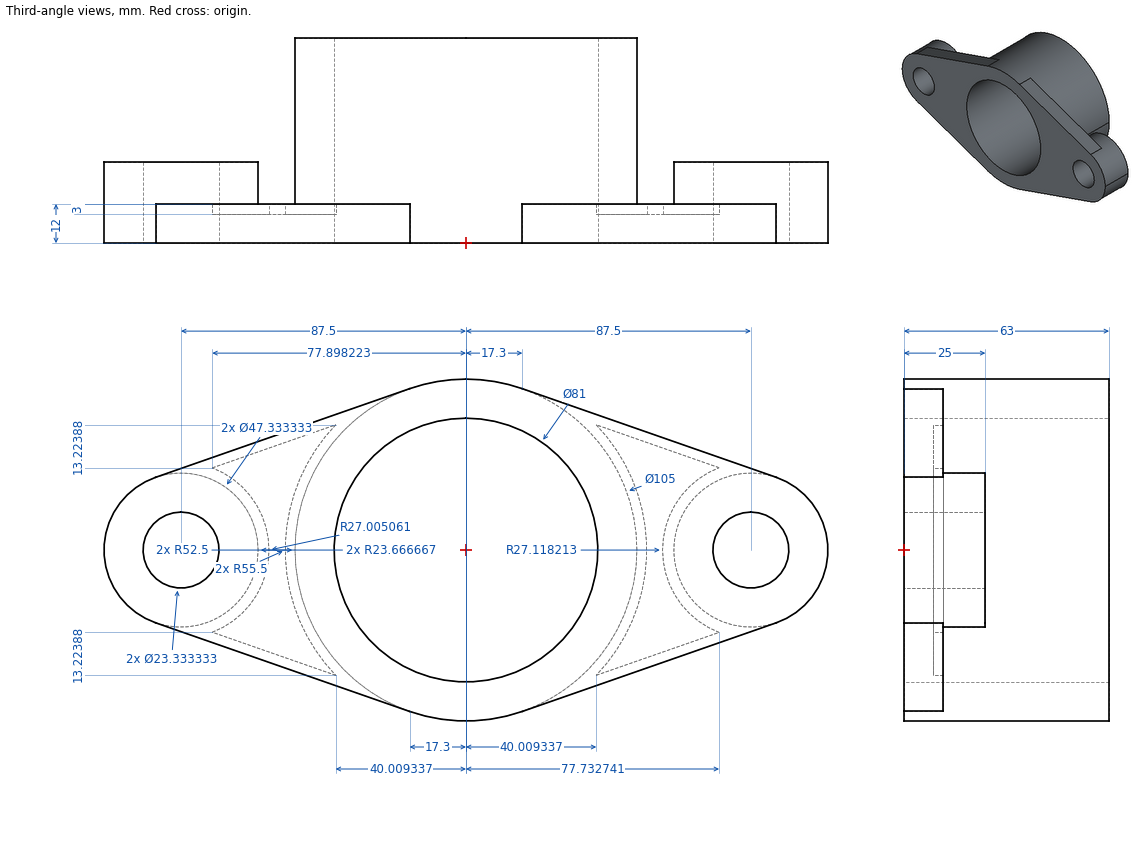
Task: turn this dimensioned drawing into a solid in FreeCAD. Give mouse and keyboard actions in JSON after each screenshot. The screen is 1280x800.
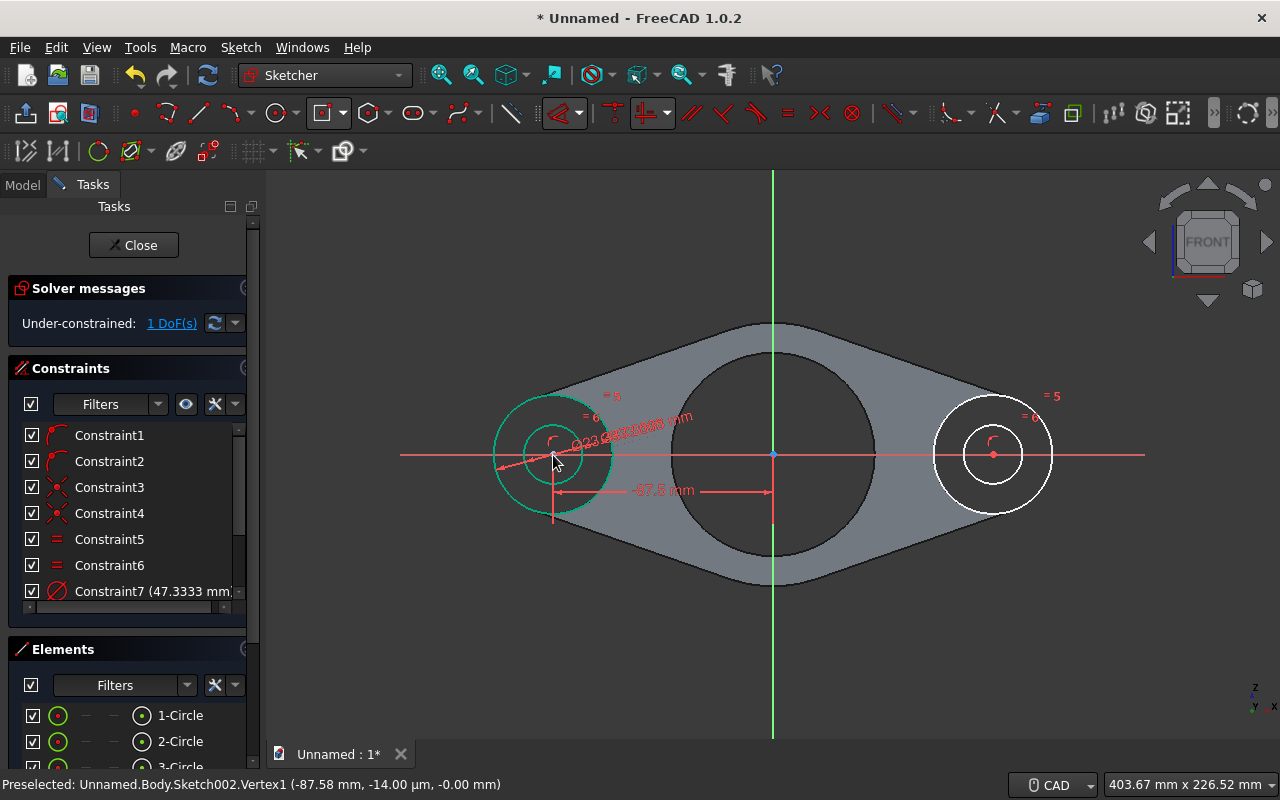
{"action": "left_click", "coordinate": [993, 455]}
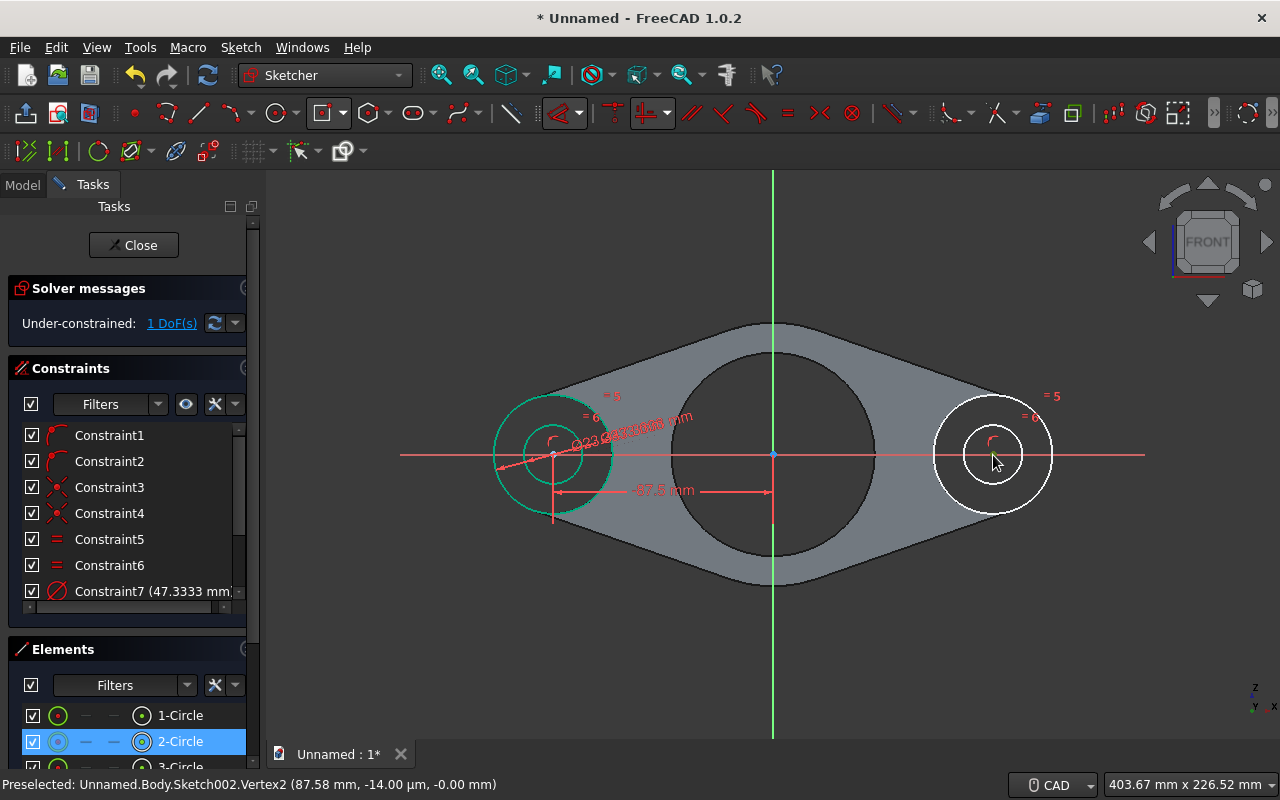
{"action": "key", "text": "l"}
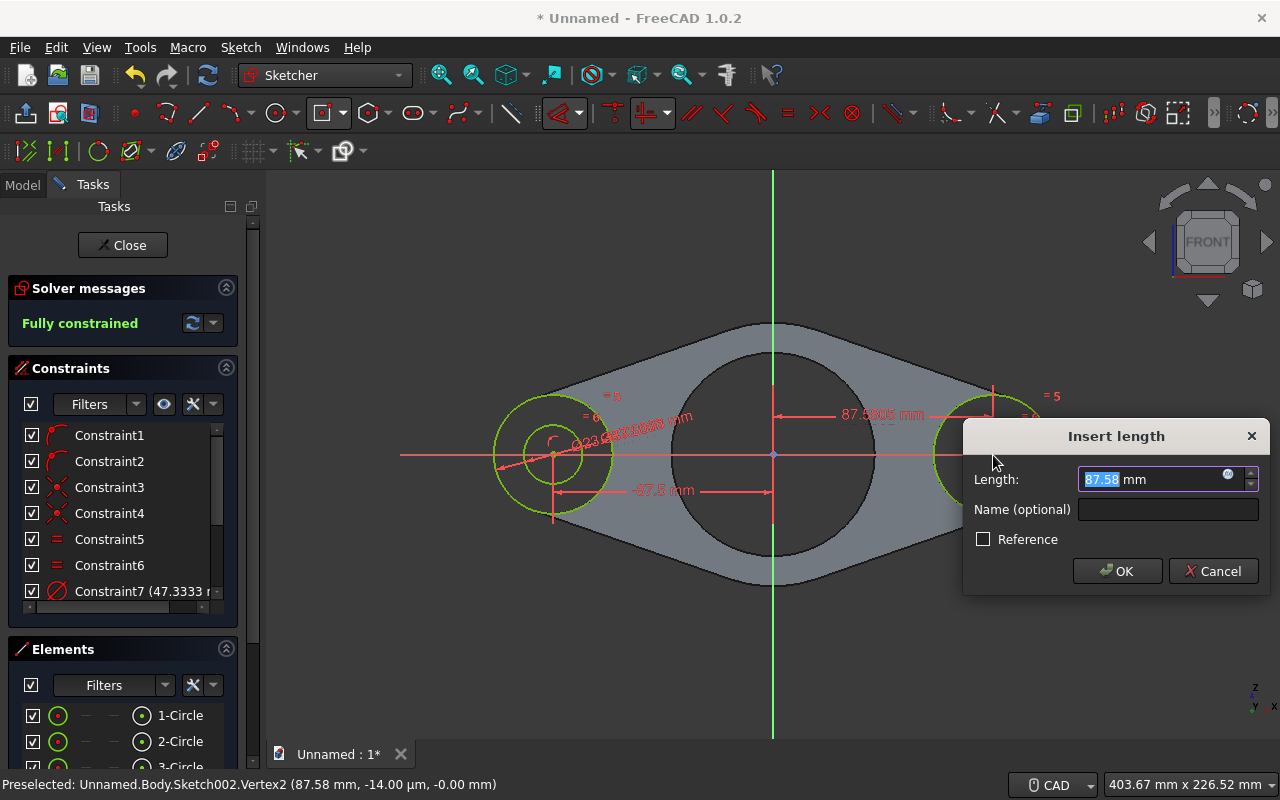
{"action": "type", "text": "87.5"}
{"action": "key", "text": "Return"}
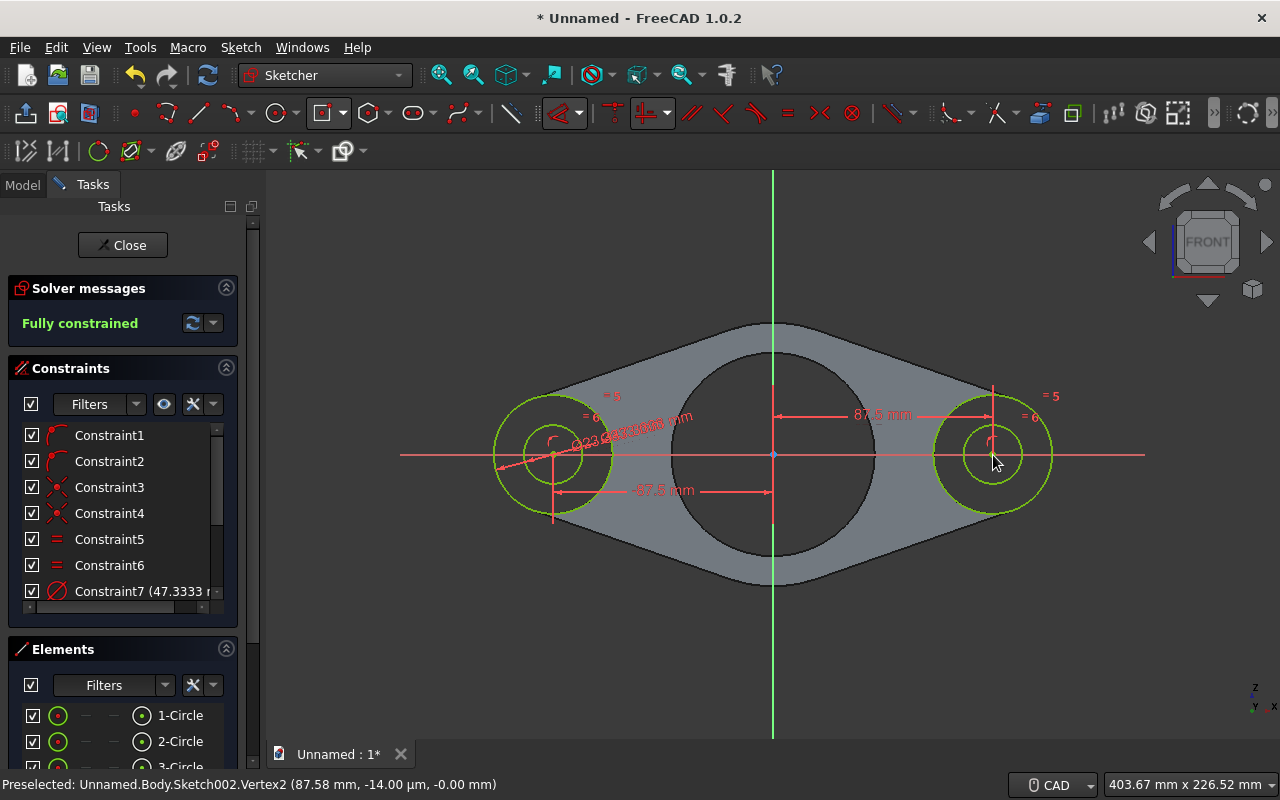
{"action": "left_click", "coordinate": [123, 245]}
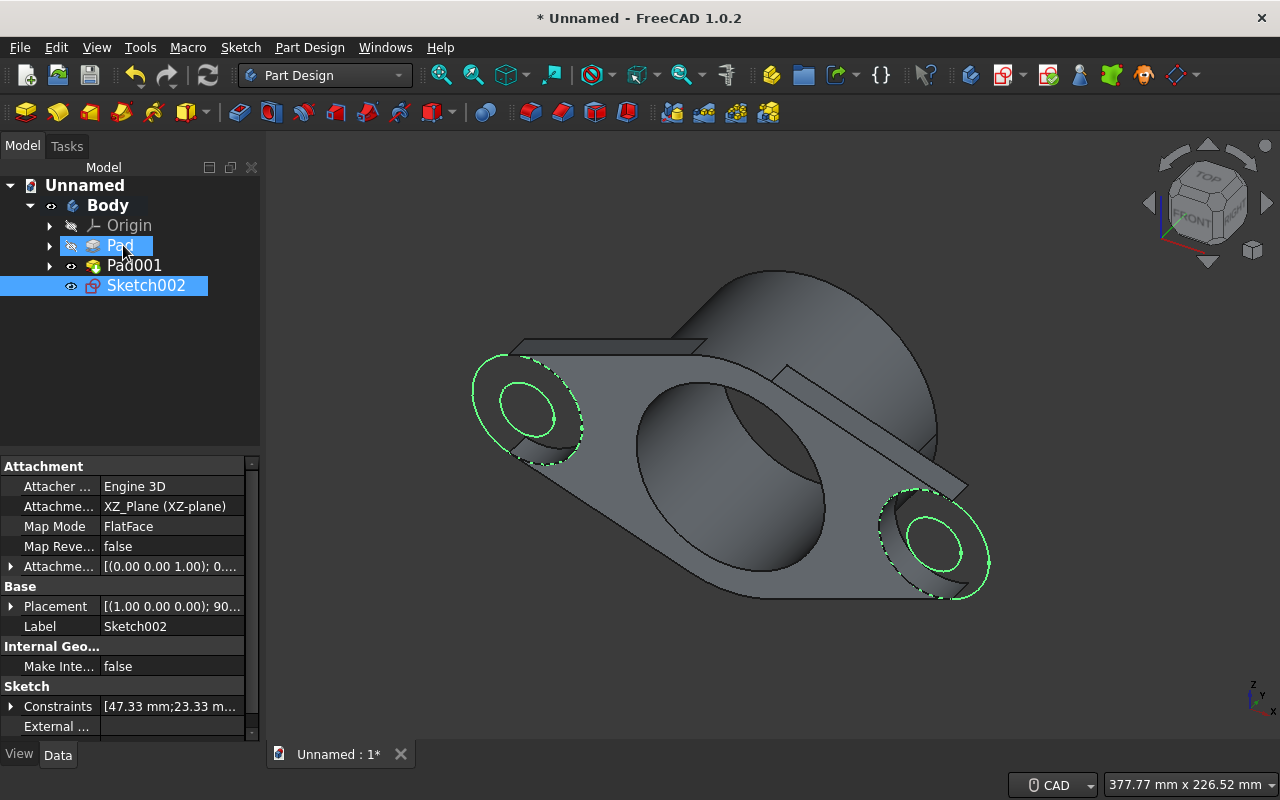
{"action": "left_click", "coordinate": [26, 112]}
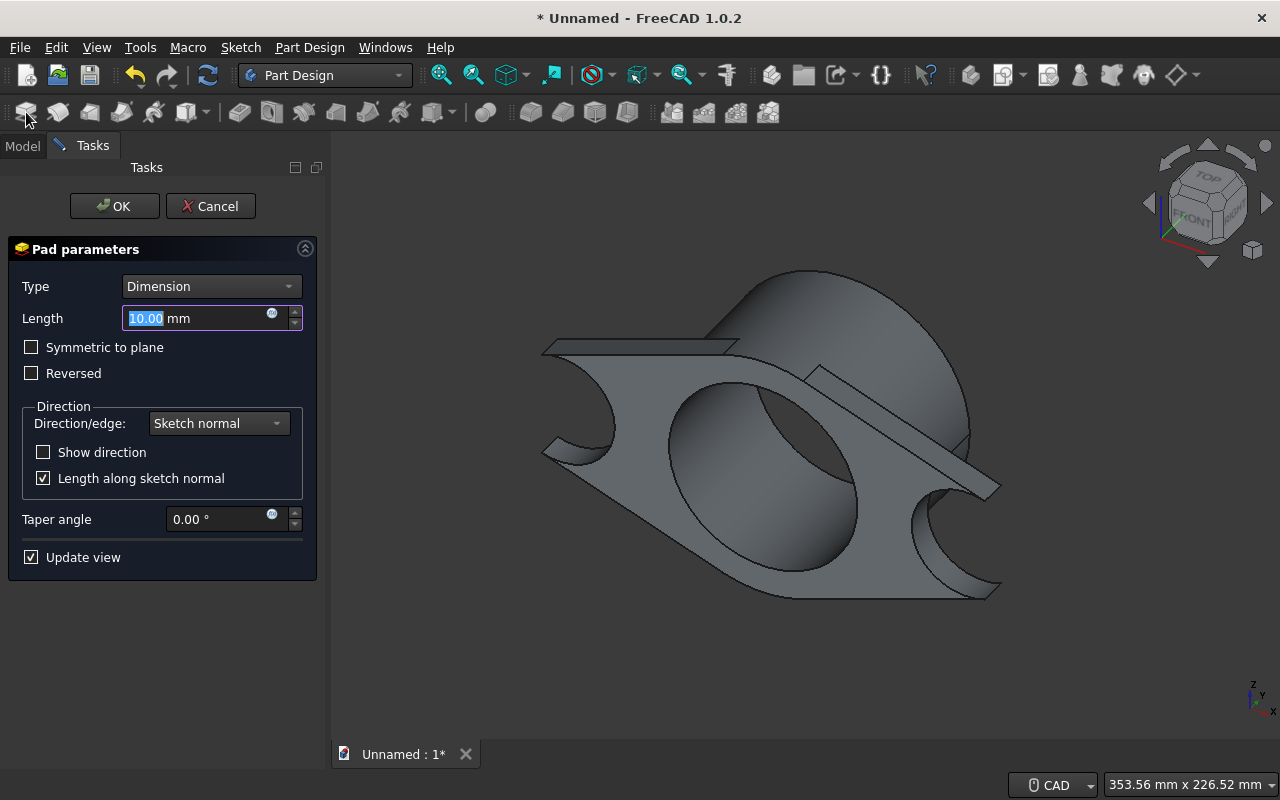
{"action": "type", "text": "25"}
{"action": "key", "text": "Tab"}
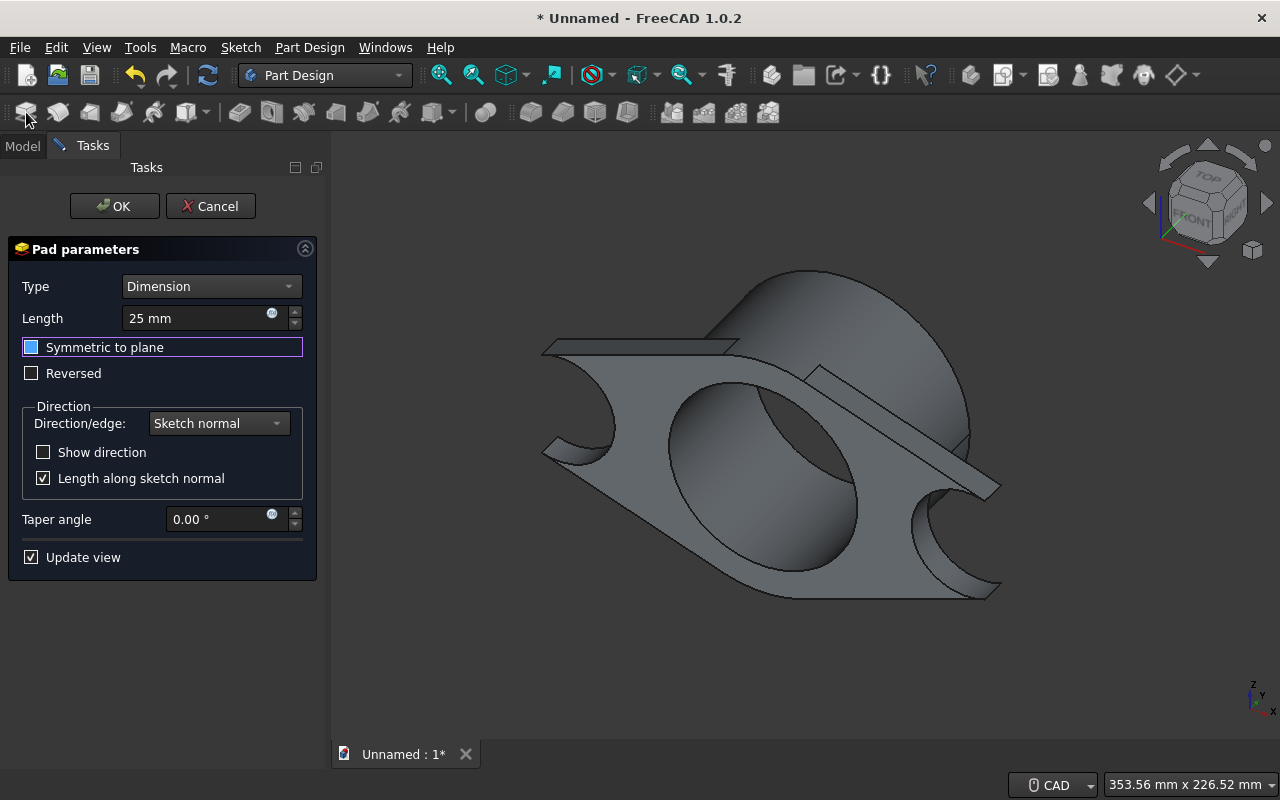
{"action": "left_click", "coordinate": [30, 373]}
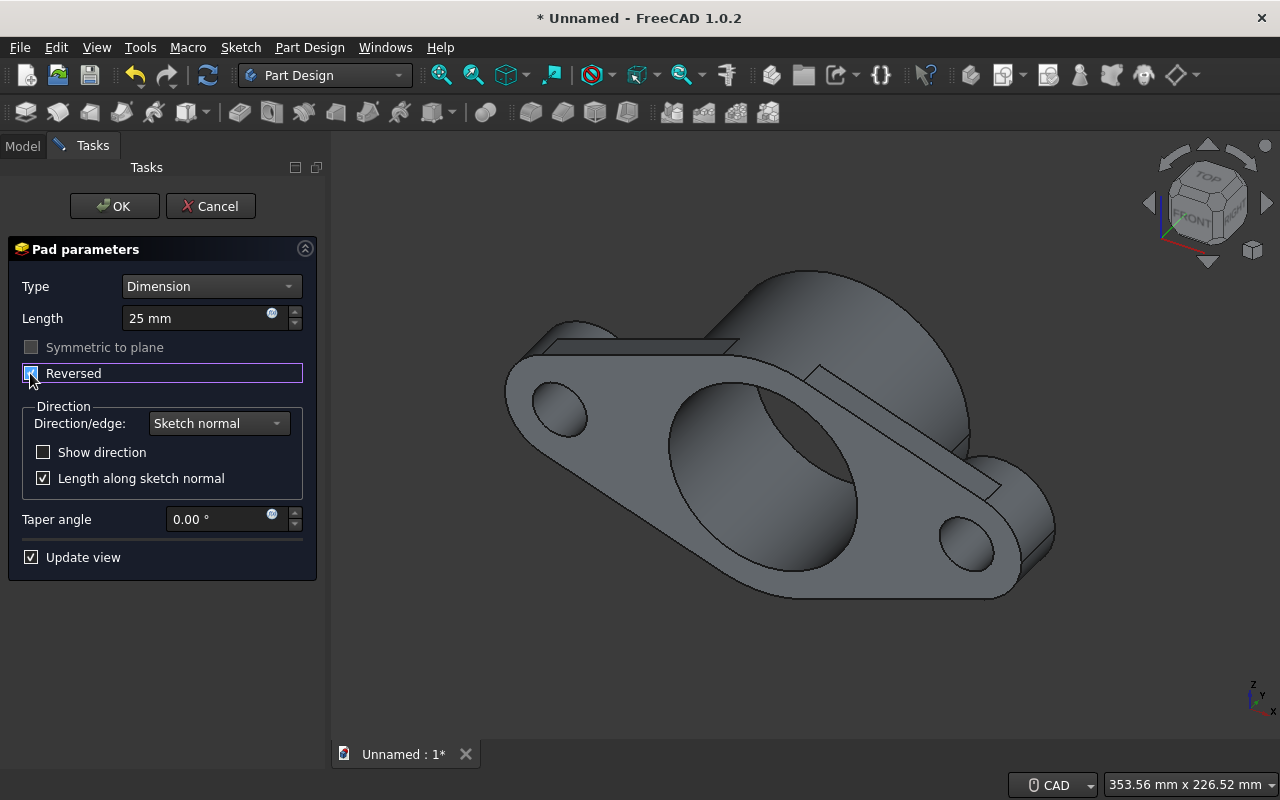
{"action": "left_click", "coordinate": [115, 206]}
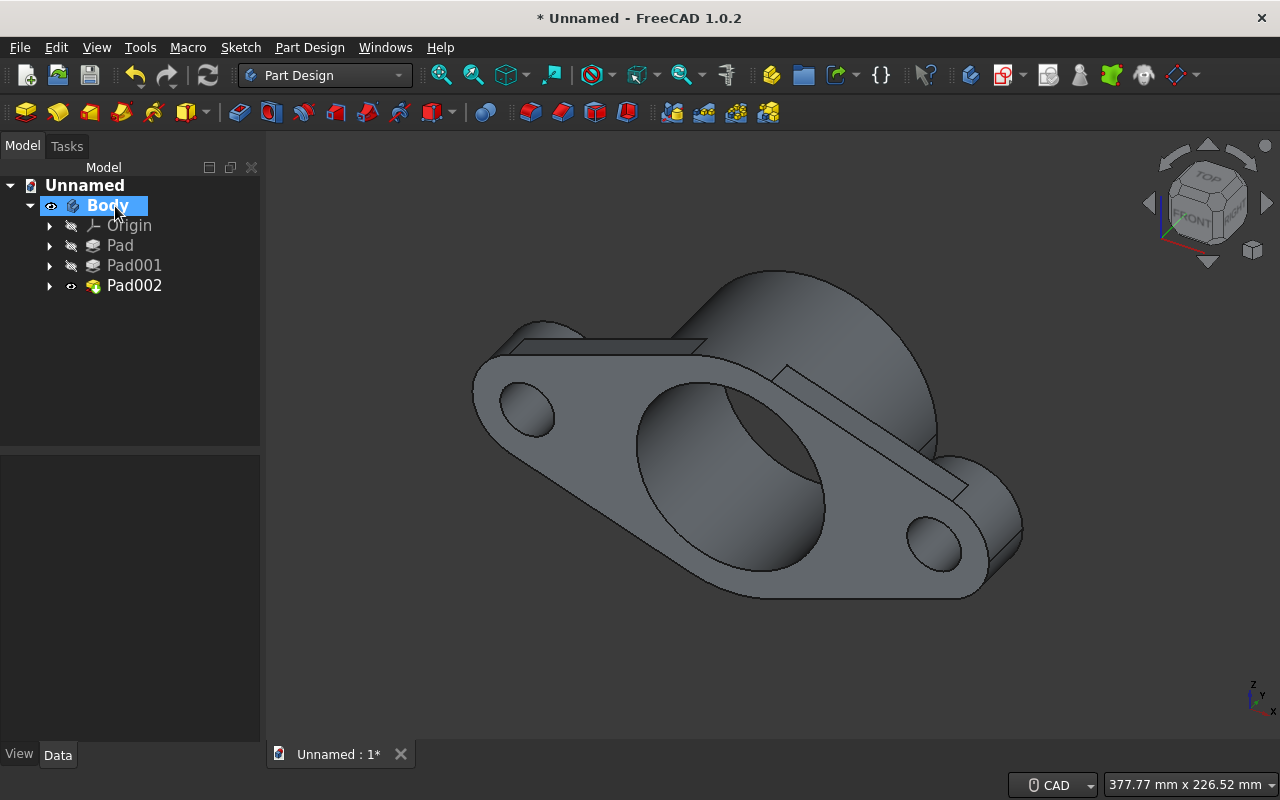
{"action": "key", "text": "4"}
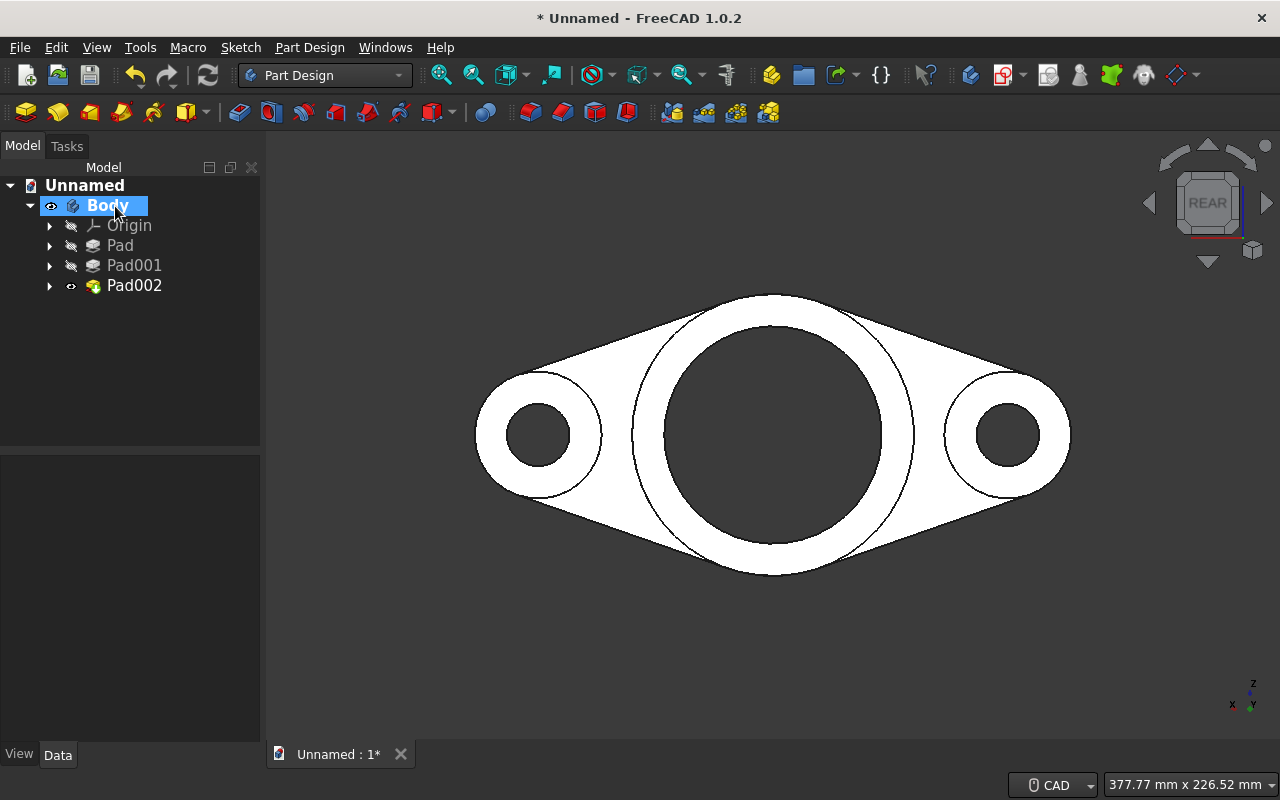
{"action": "left_click", "coordinate": [622, 358]}